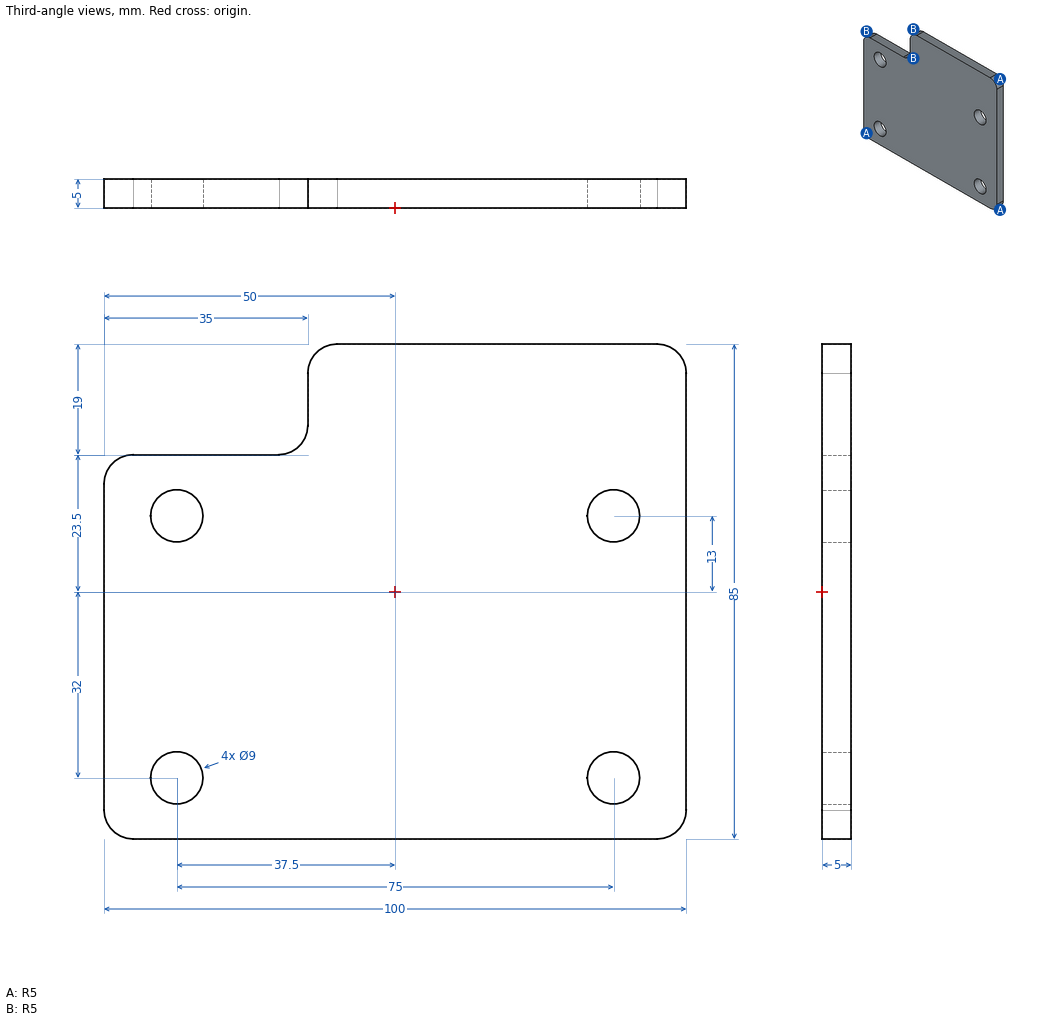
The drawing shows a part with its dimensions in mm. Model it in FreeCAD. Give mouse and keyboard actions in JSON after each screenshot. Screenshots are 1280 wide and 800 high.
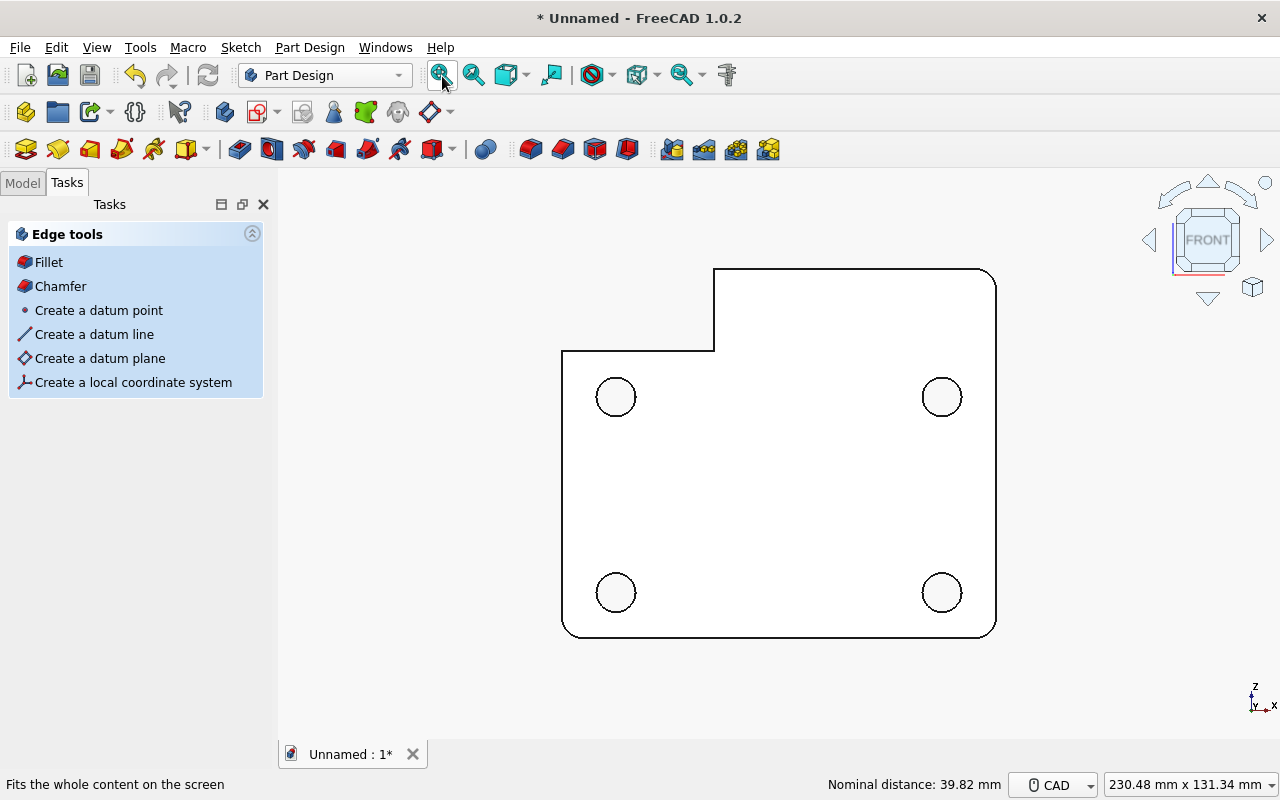
{"action": "scroll", "coordinate": [714, 350], "scroll_direction": "up", "scroll_amount": 4}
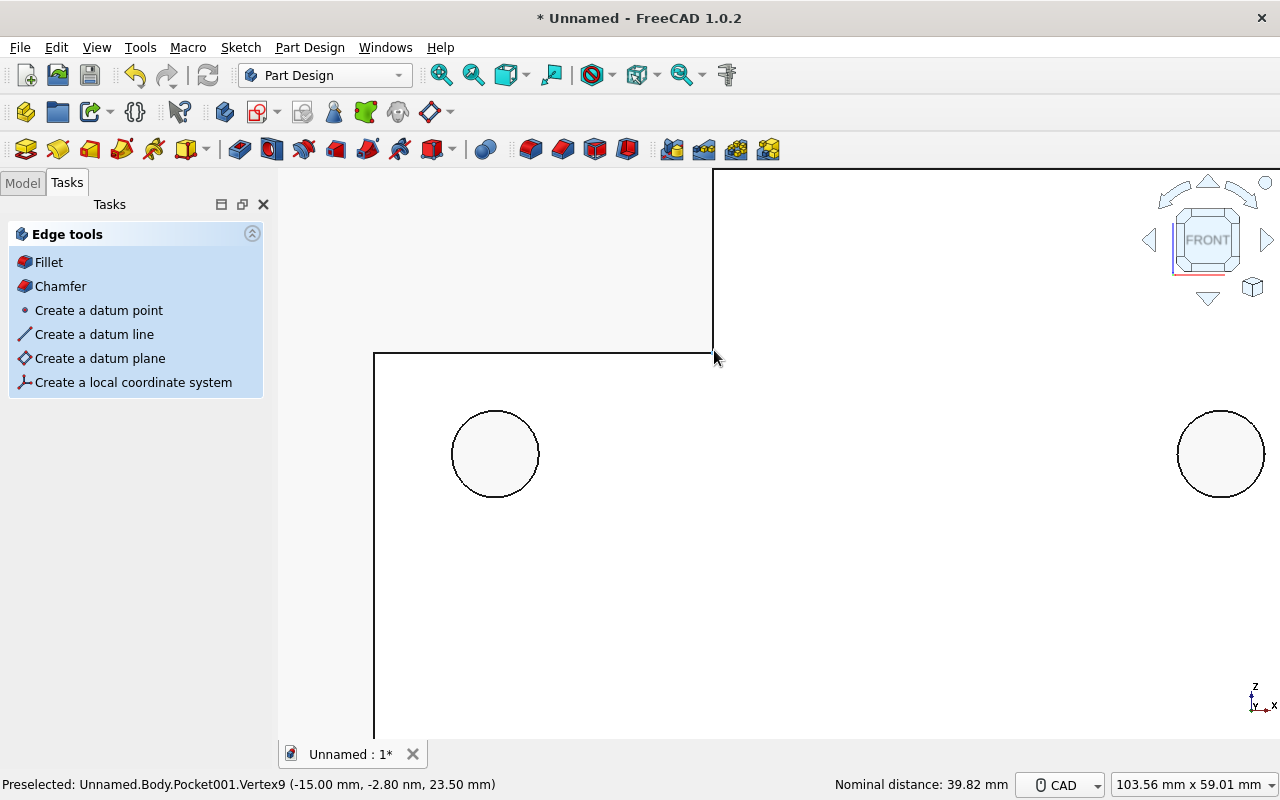
{"action": "left_click", "coordinate": [442, 76]}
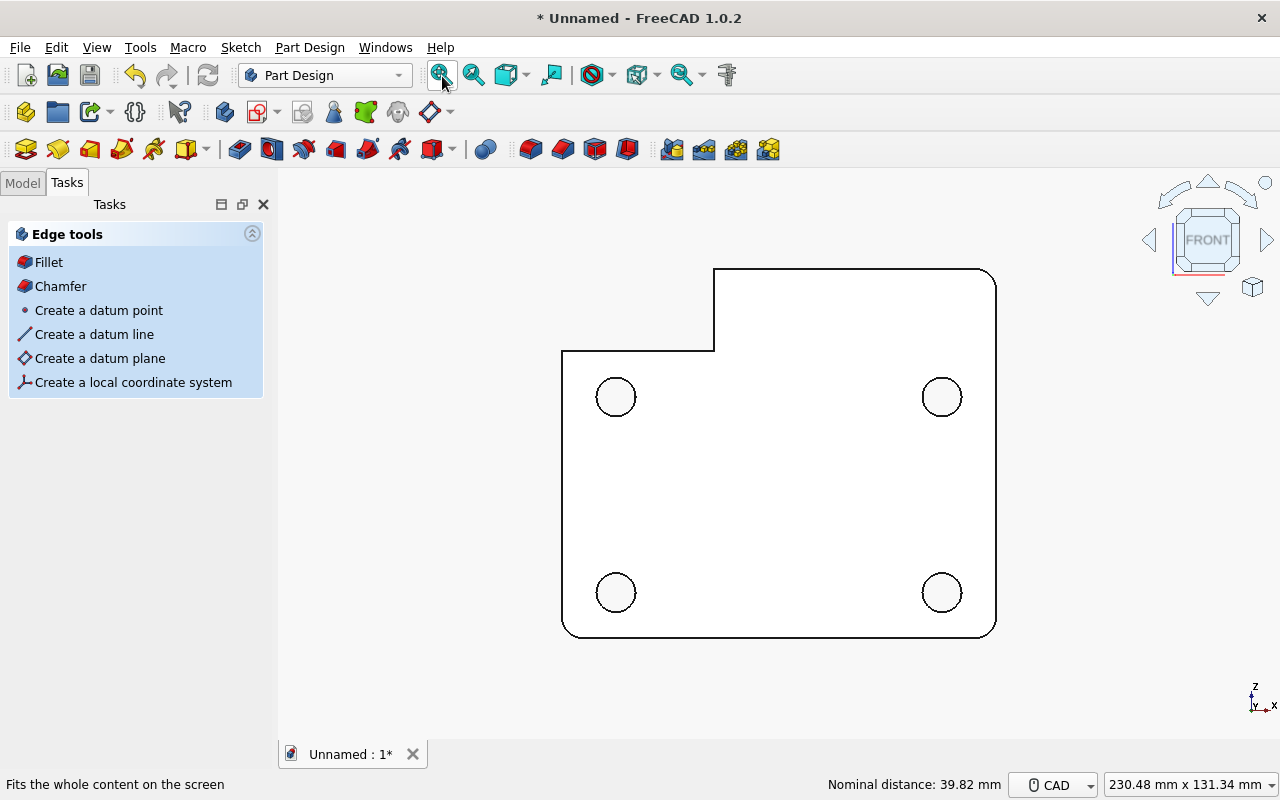
{"action": "key", "text": "3"}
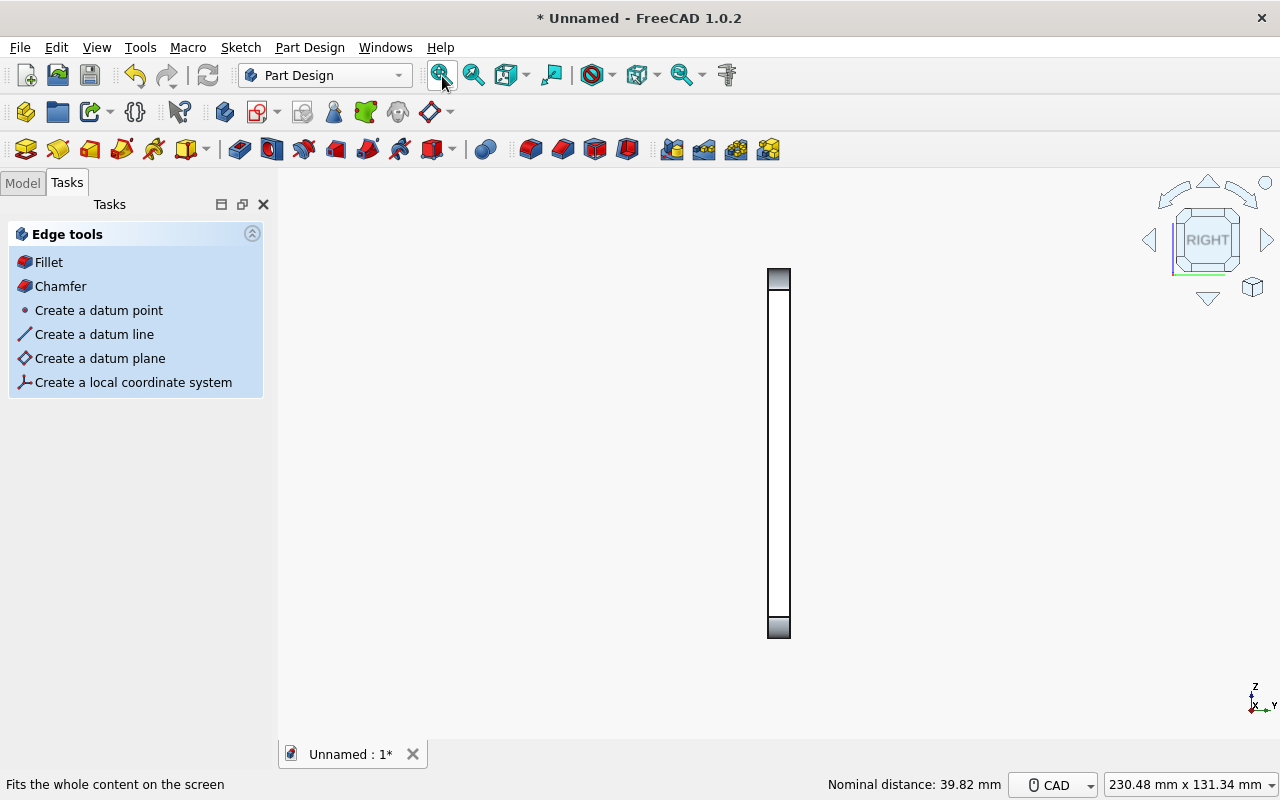
{"action": "scroll", "coordinate": [779, 350], "scroll_direction": "up", "scroll_amount": 4}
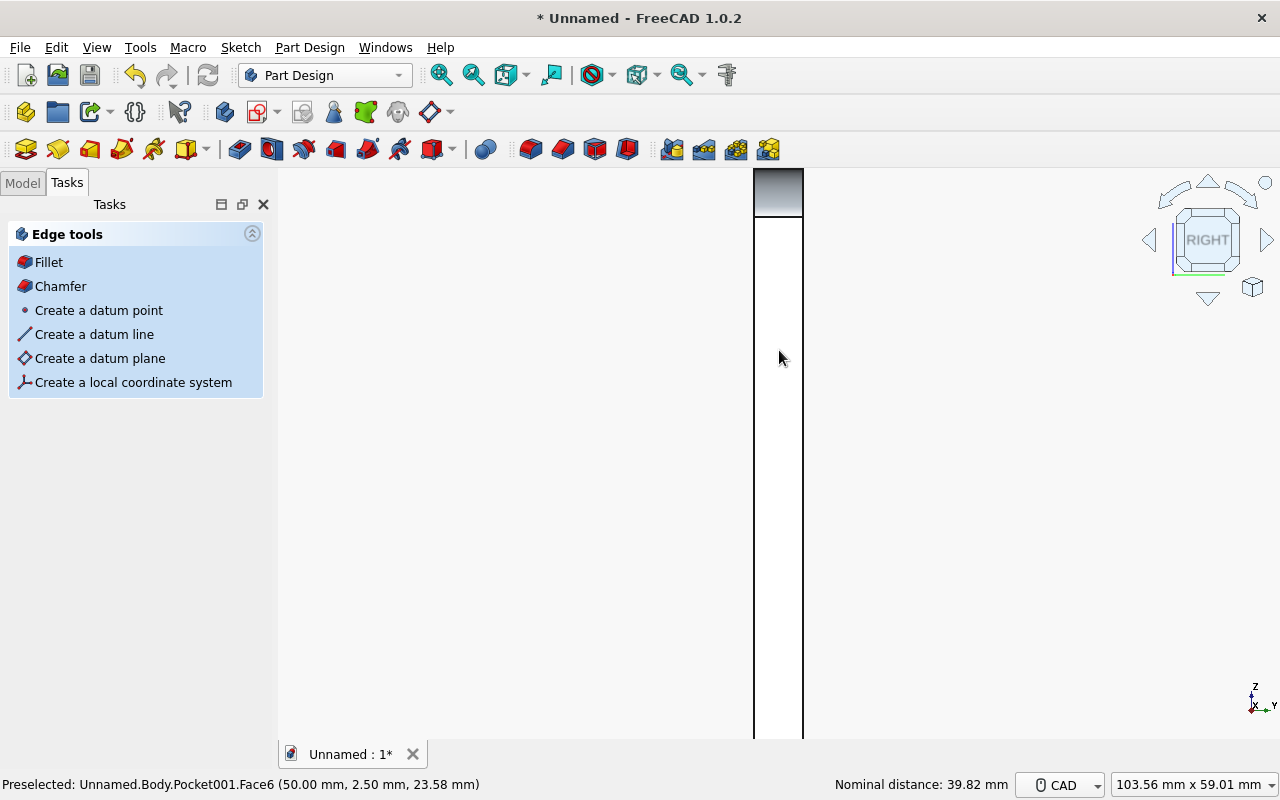
{"action": "left_click", "coordinate": [442, 76]}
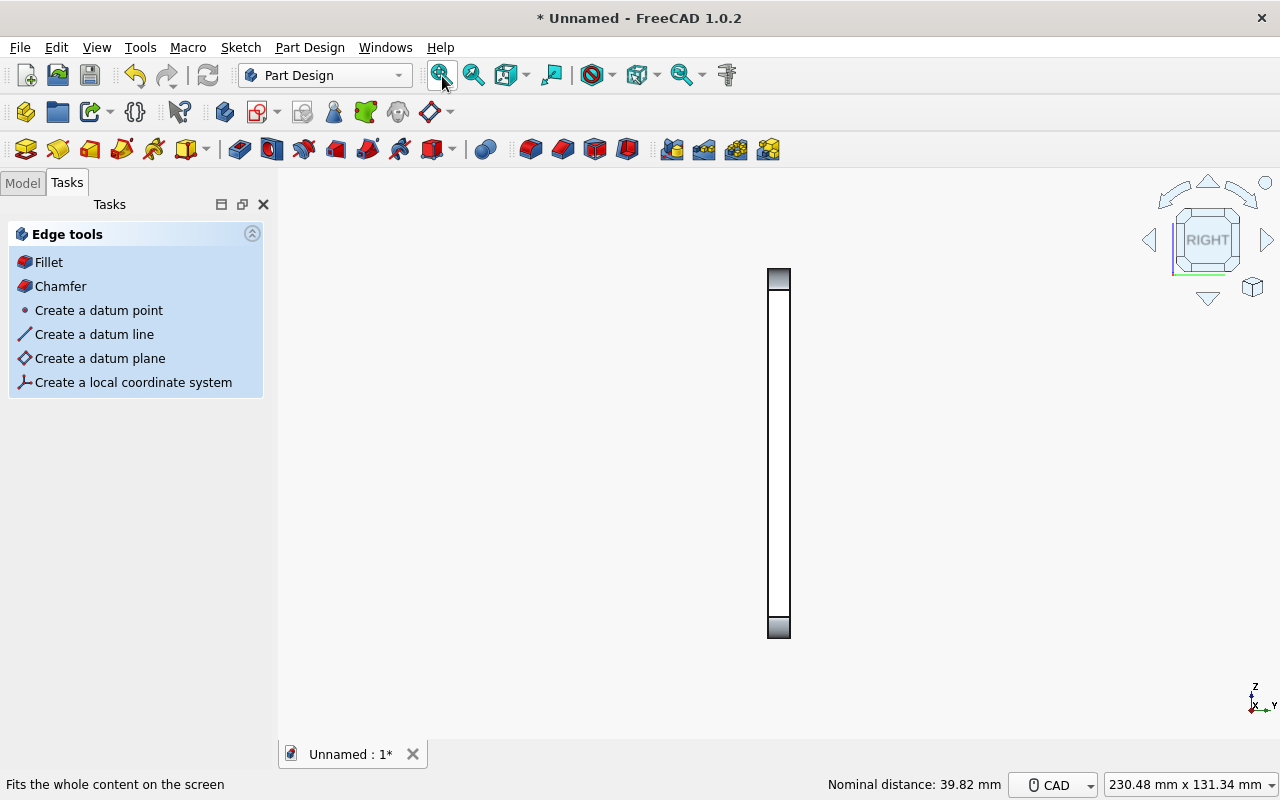
{"action": "key", "text": "5"}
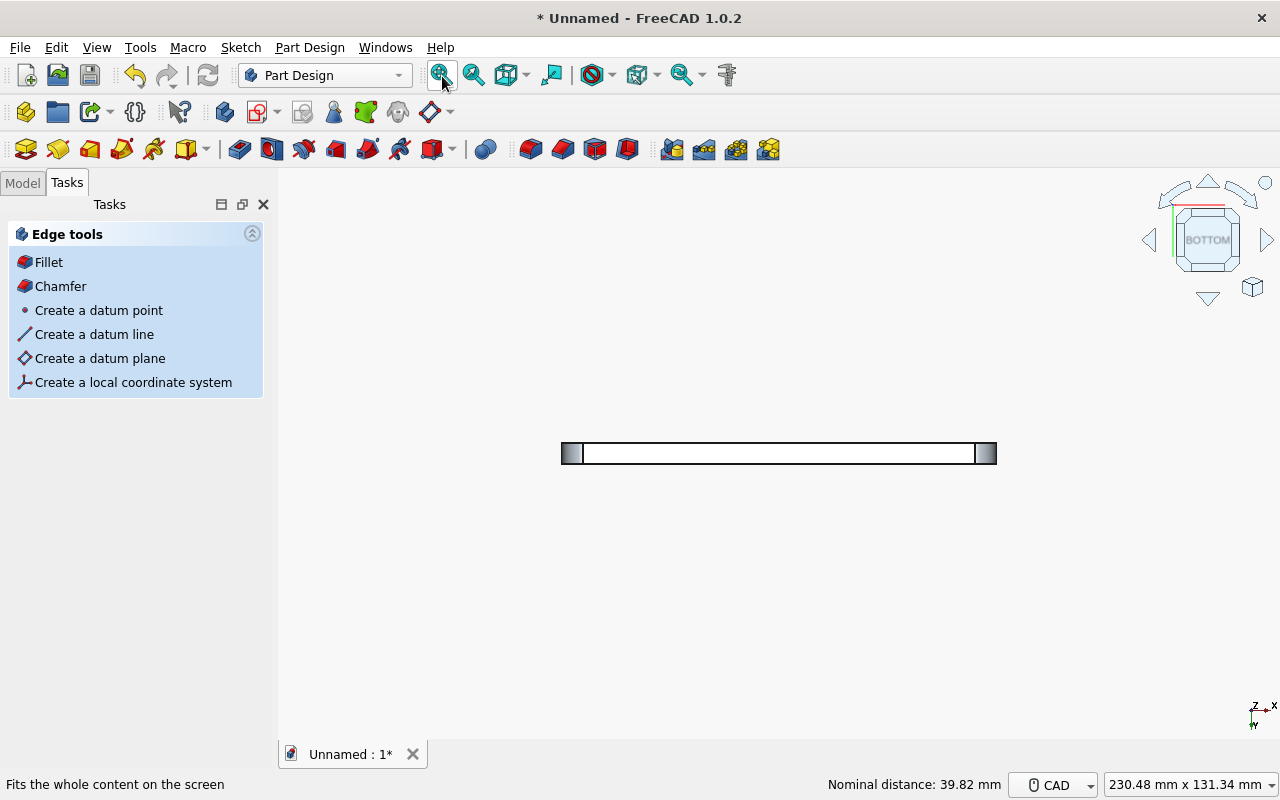
{"action": "left_click", "coordinate": [442, 76]}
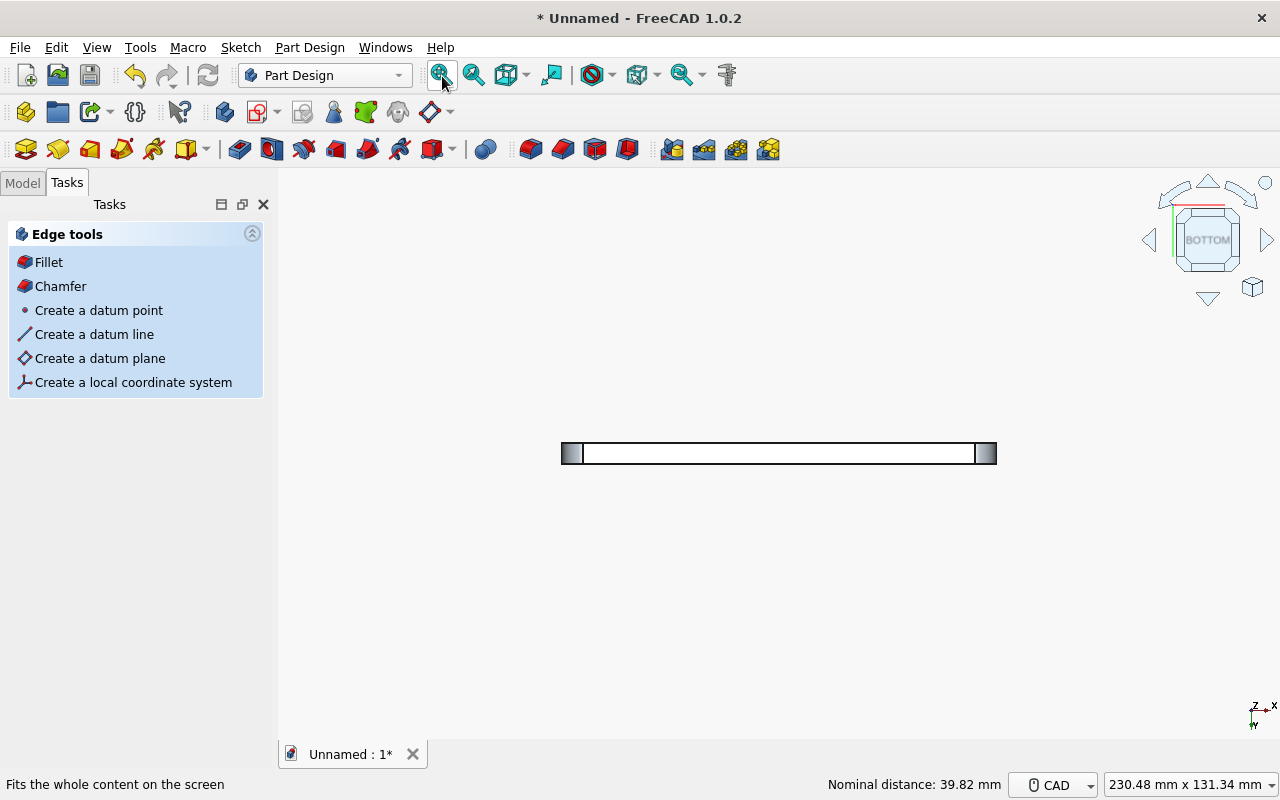
{"action": "scroll", "coordinate": [714, 452], "scroll_direction": "up", "scroll_amount": 4}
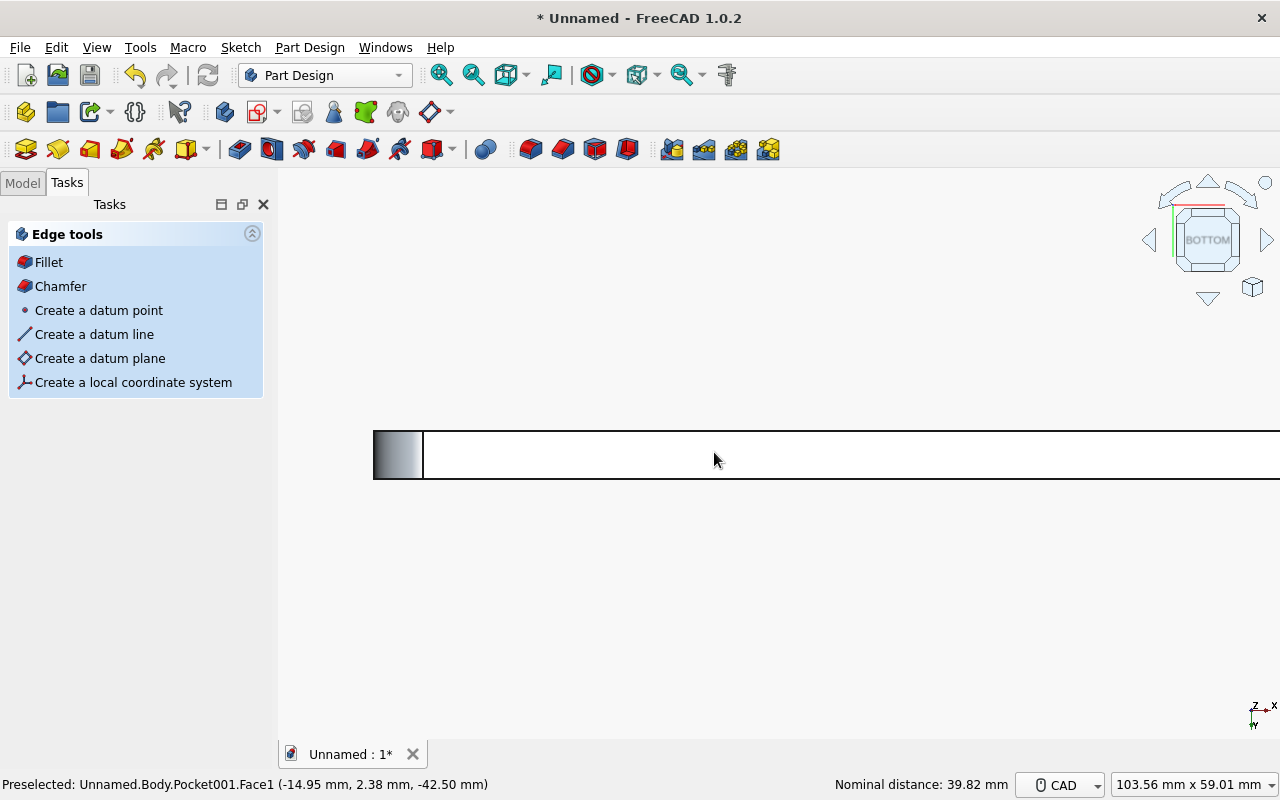
{"action": "left_click", "coordinate": [442, 76]}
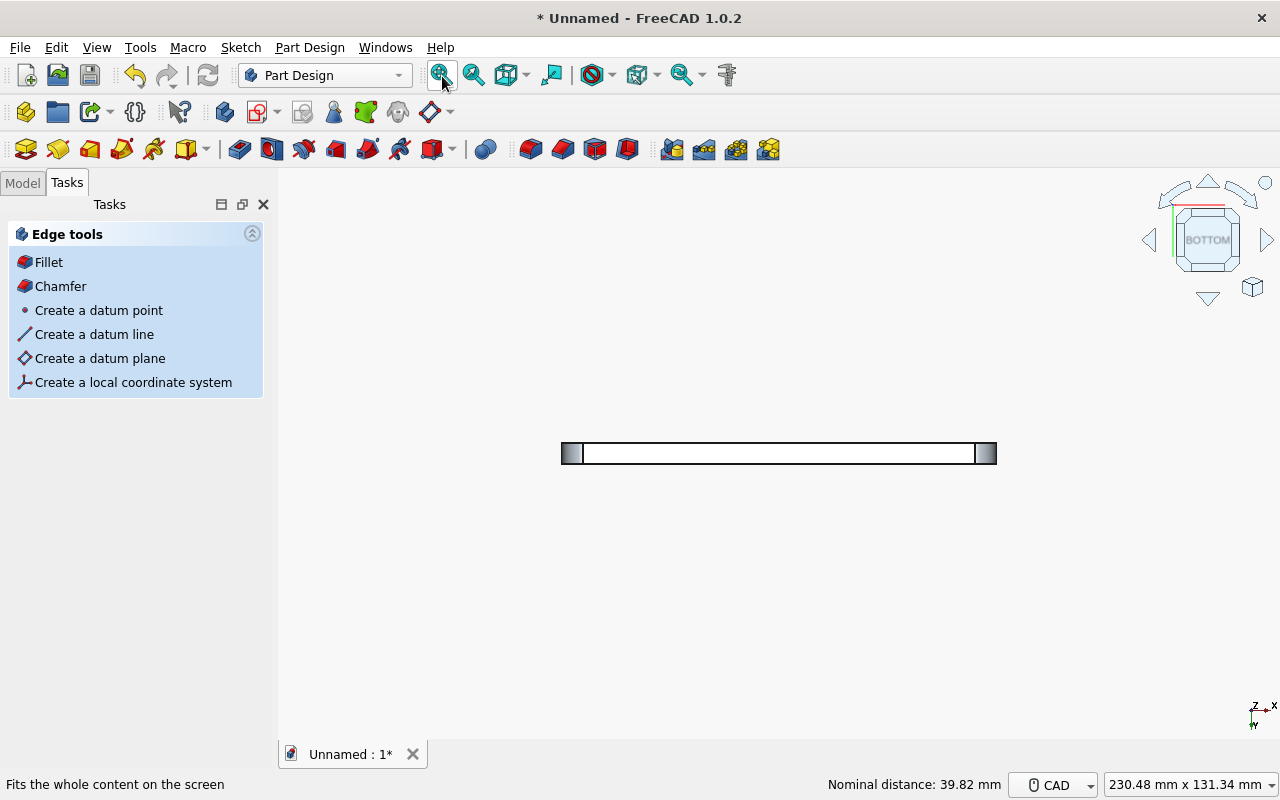
{"action": "key", "text": "4"}